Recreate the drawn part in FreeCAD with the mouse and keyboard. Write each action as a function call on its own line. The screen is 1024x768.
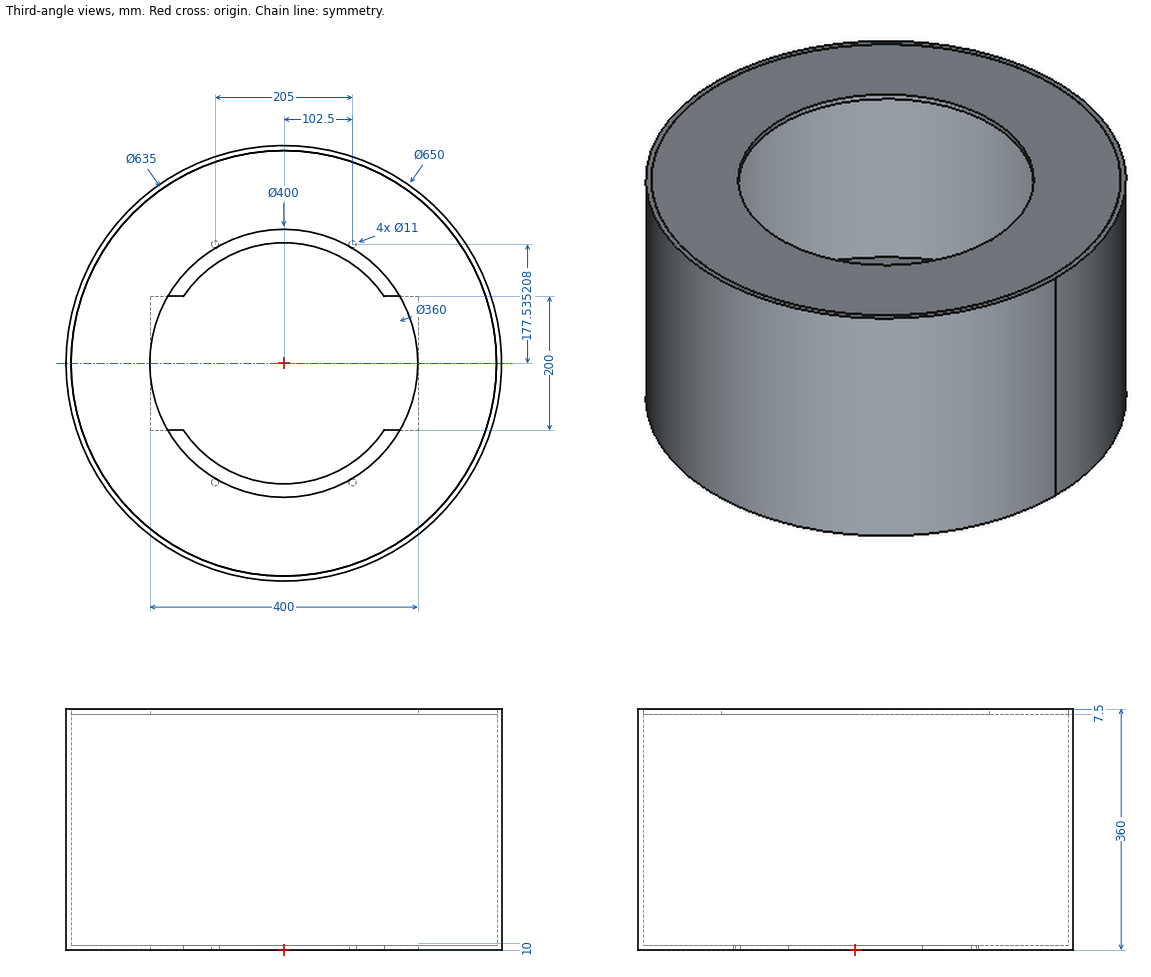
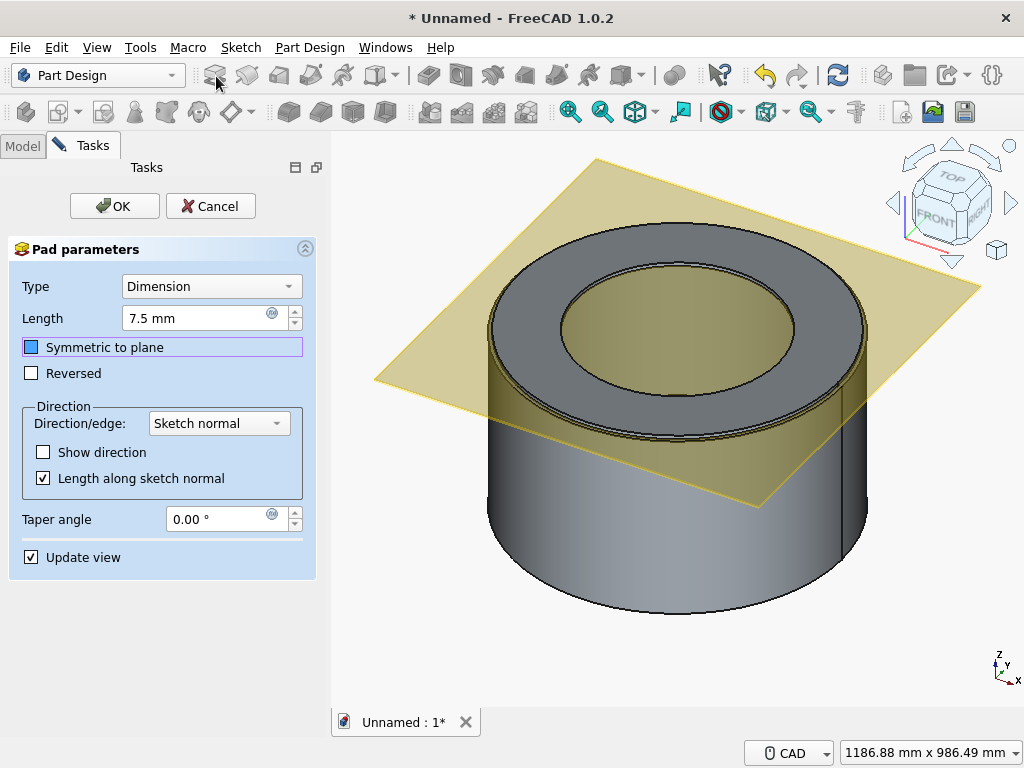
click(30, 373)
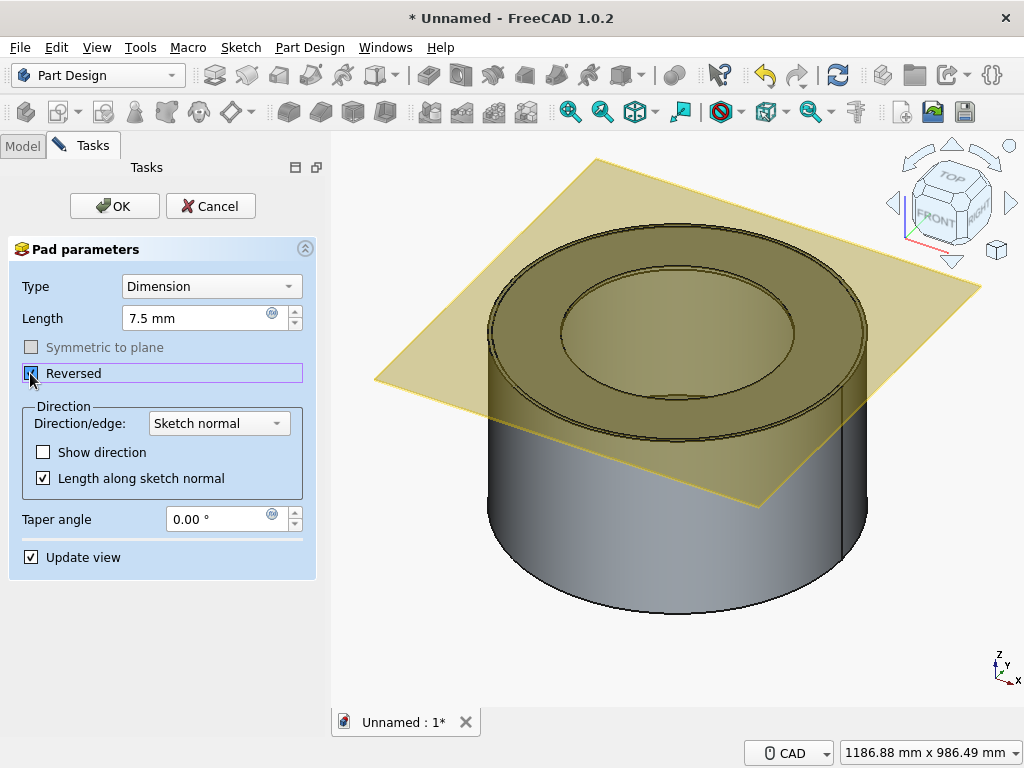
click(115, 206)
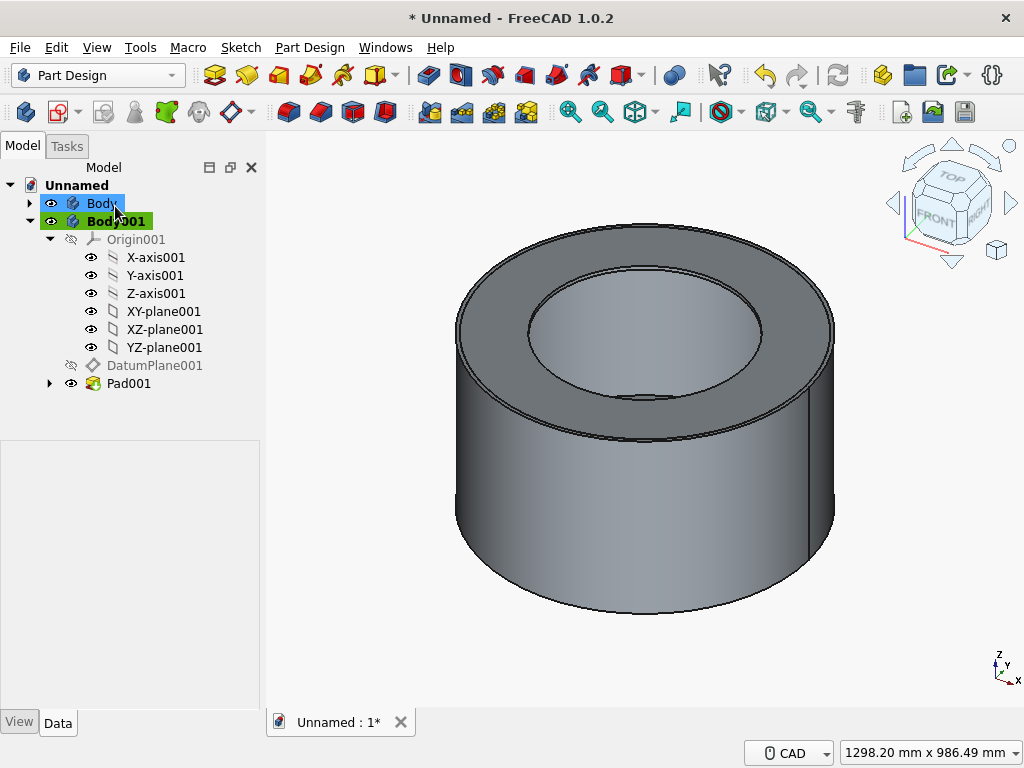
key(0)